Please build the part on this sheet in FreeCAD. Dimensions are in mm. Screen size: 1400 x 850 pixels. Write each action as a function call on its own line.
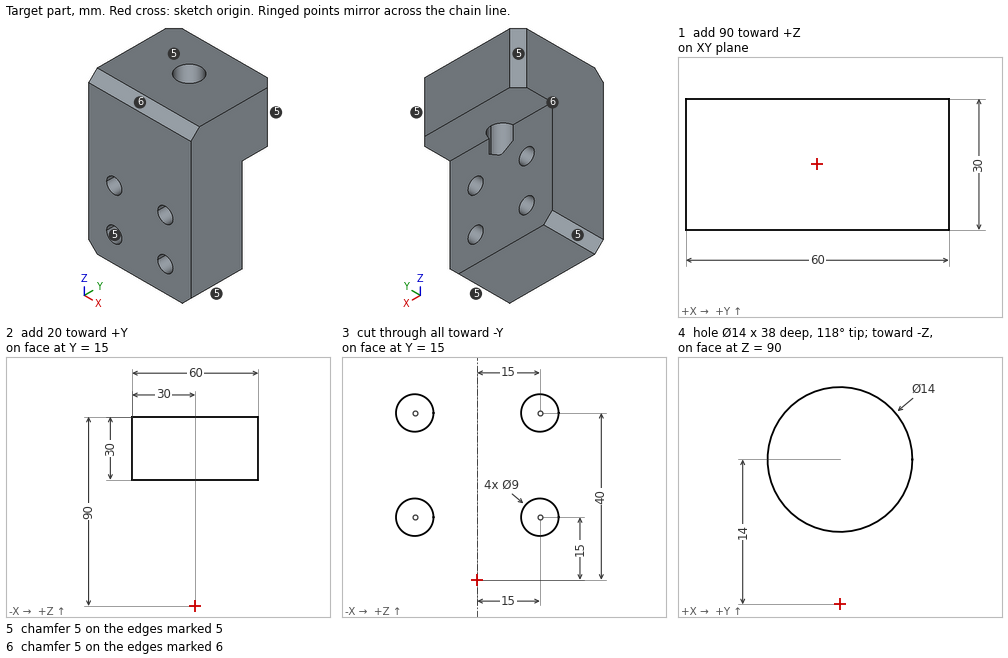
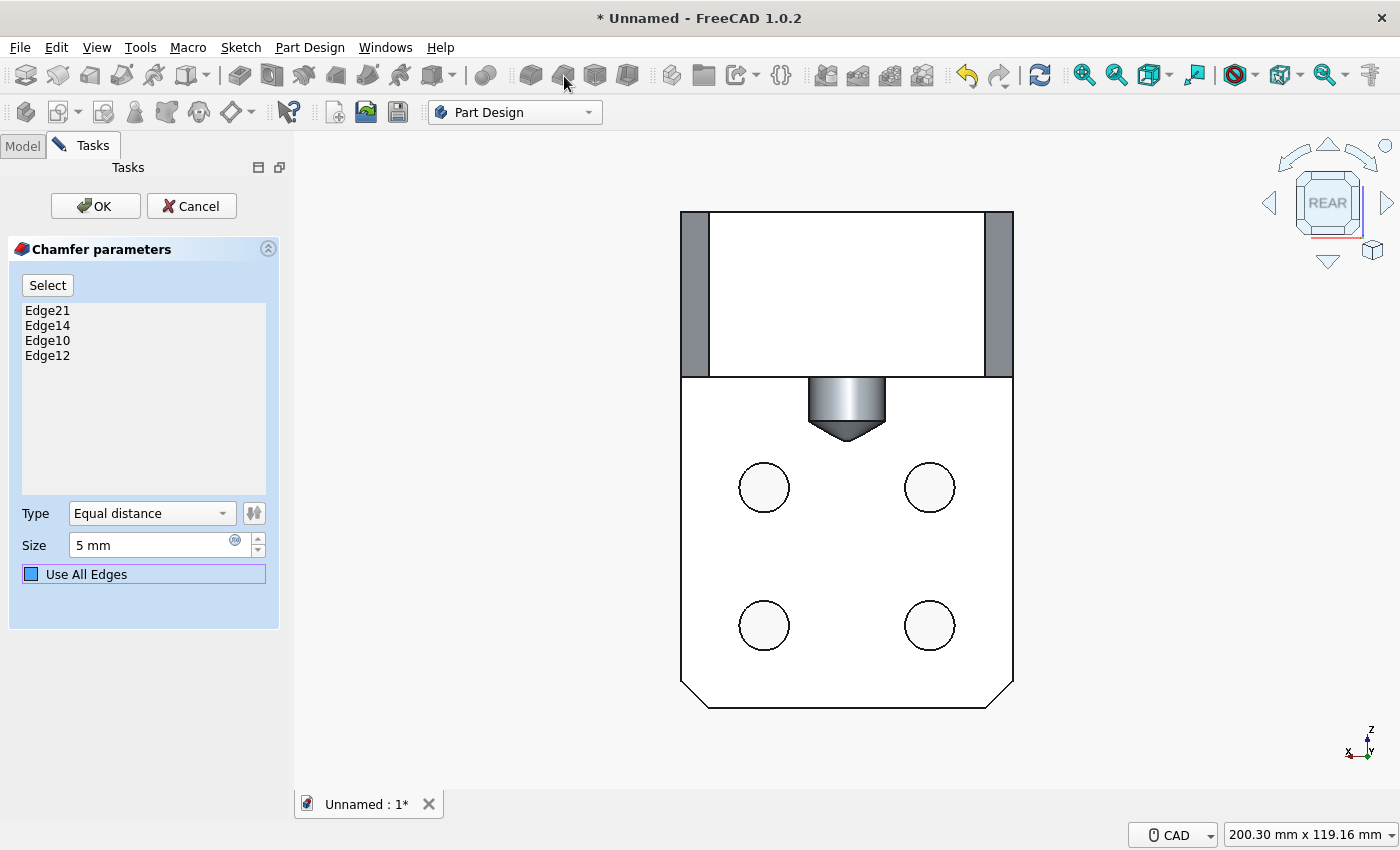
click(96, 206)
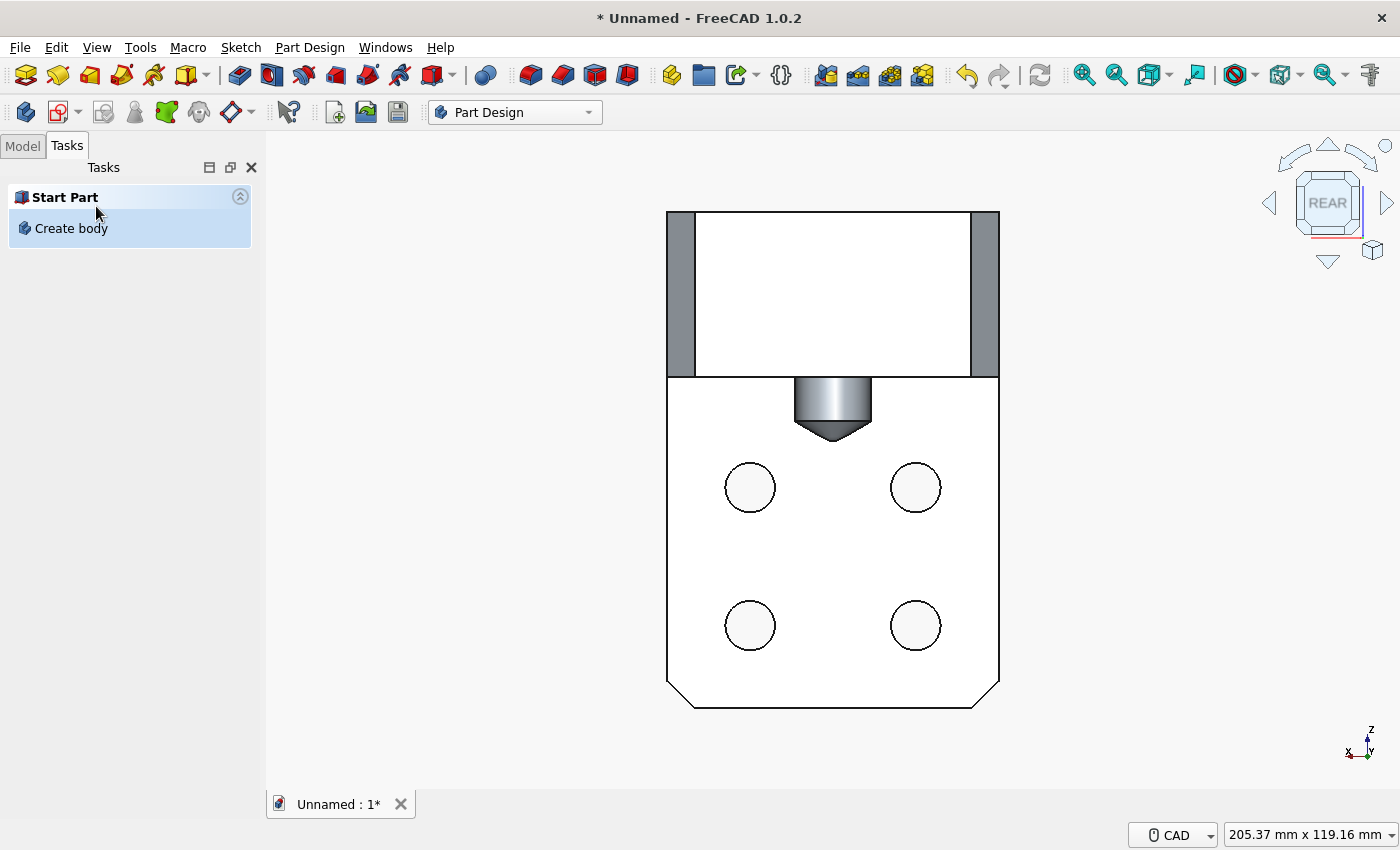
key(0)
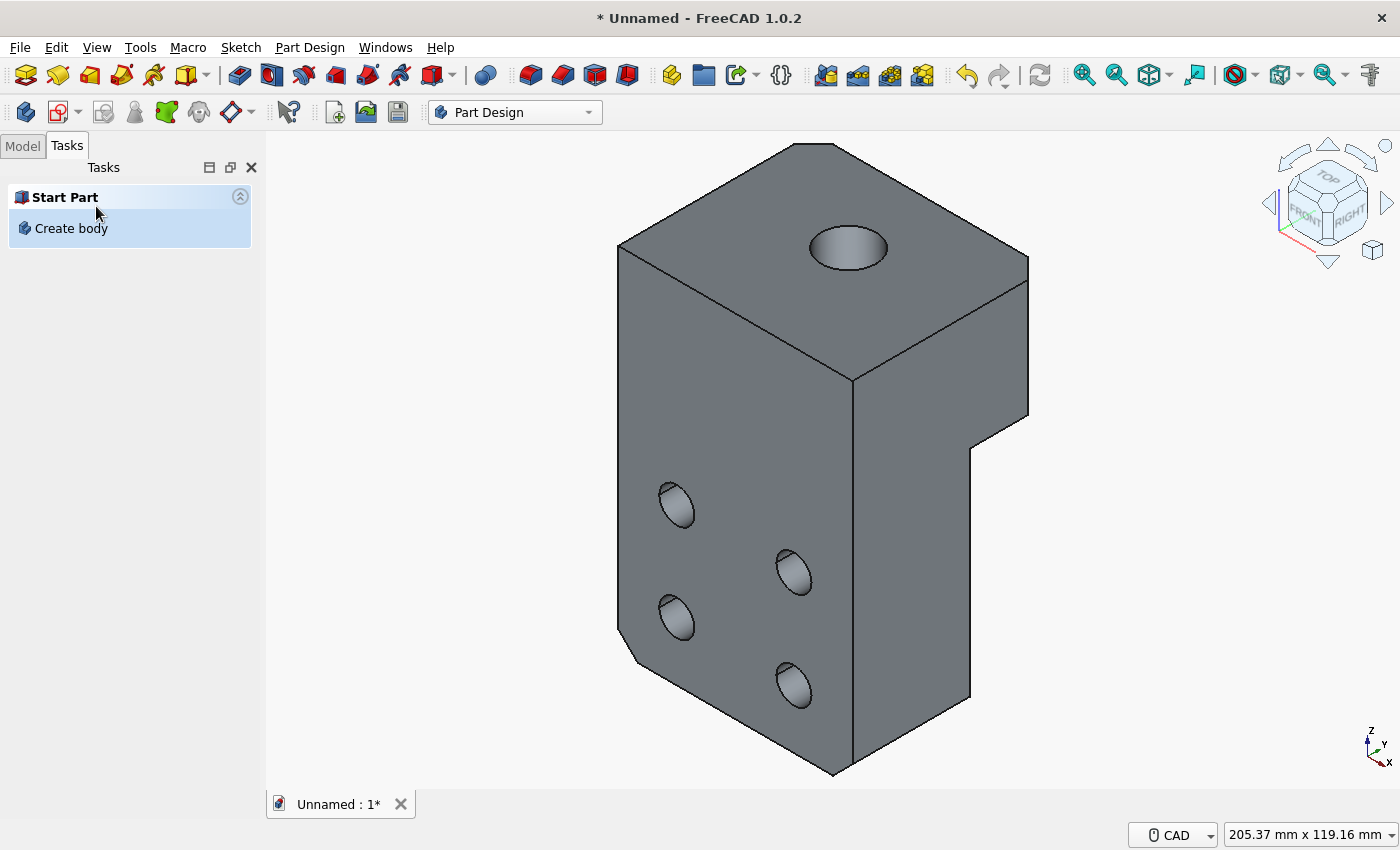
click(735, 312)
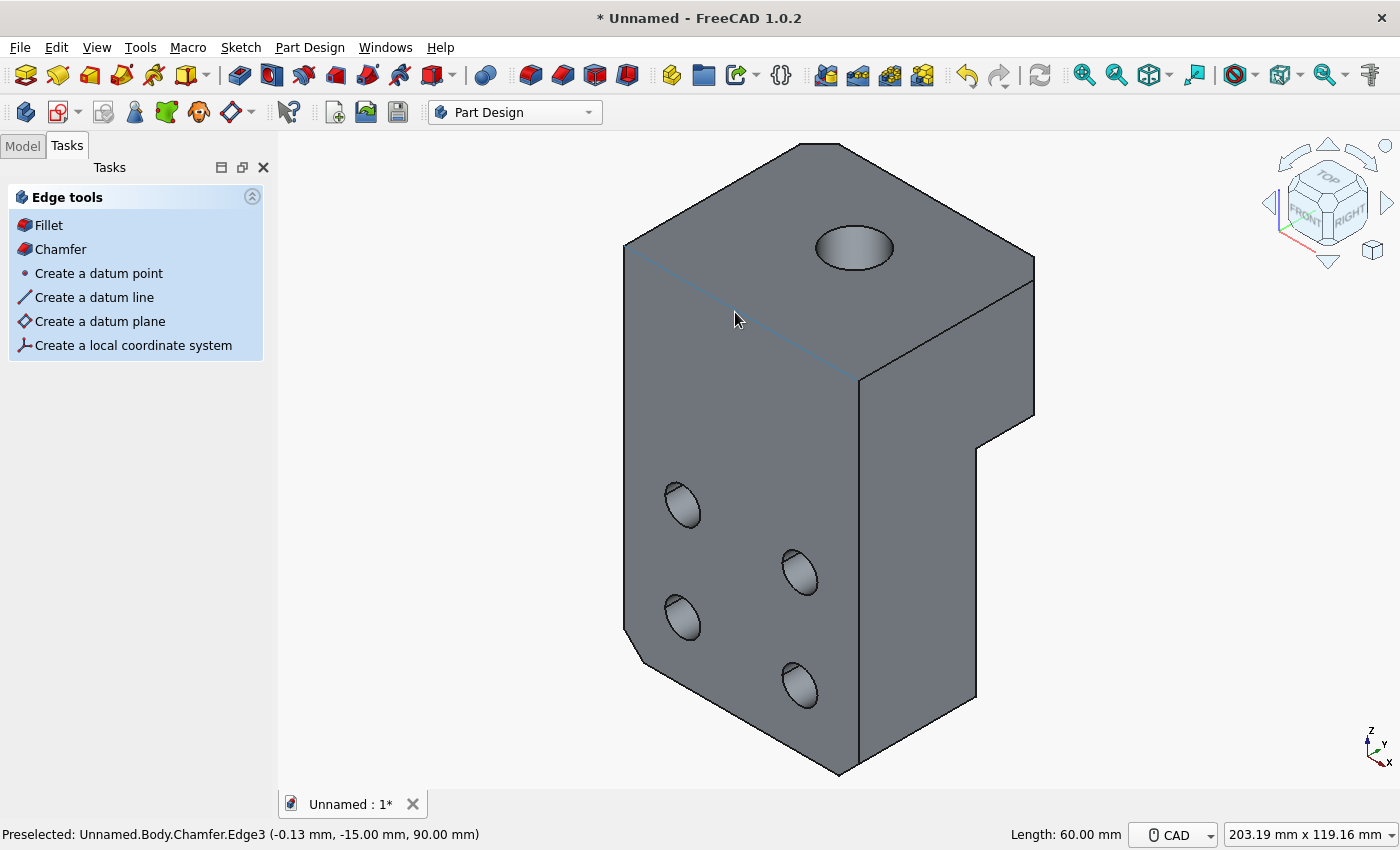
click(564, 76)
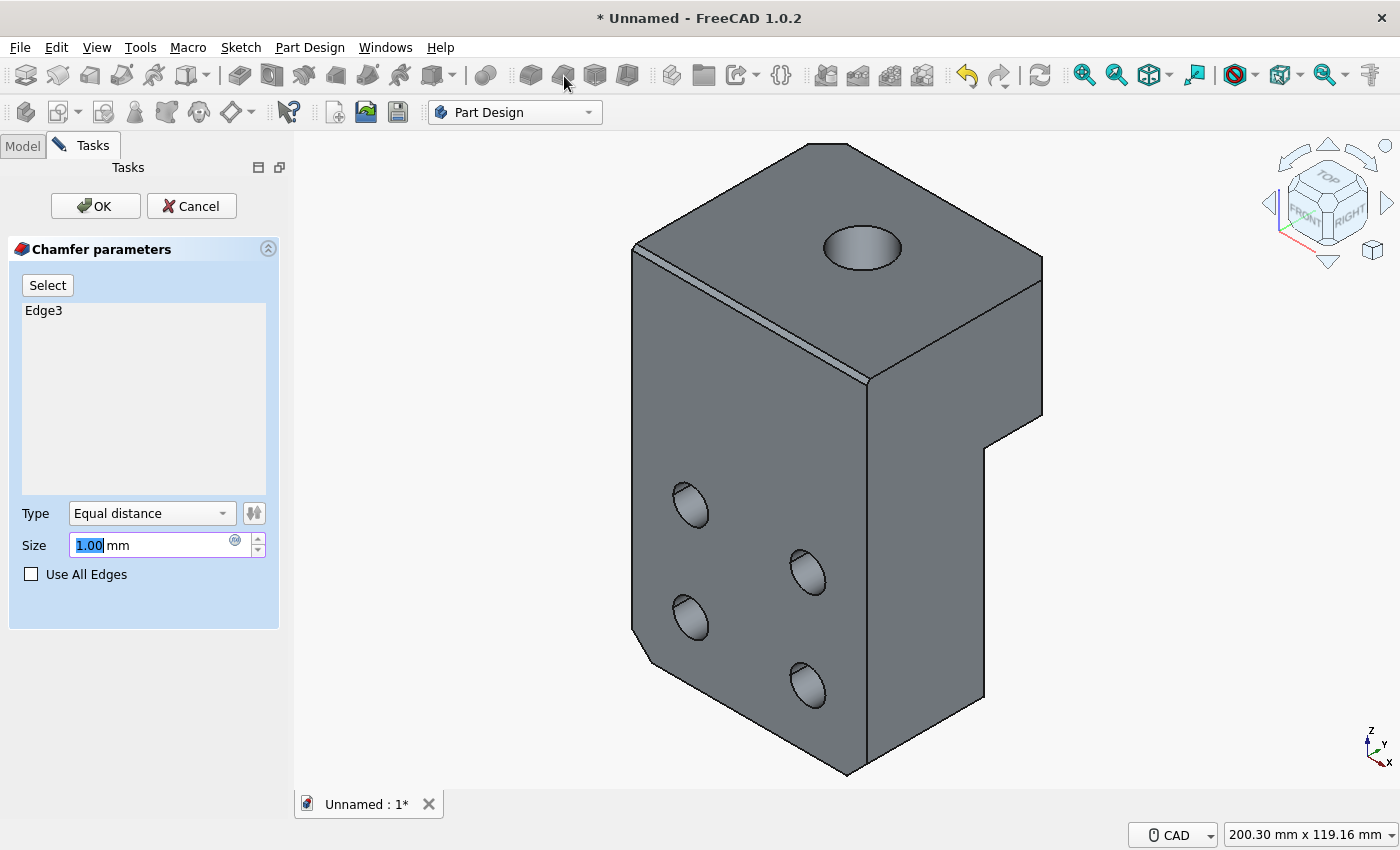
text(5)
key(Tab)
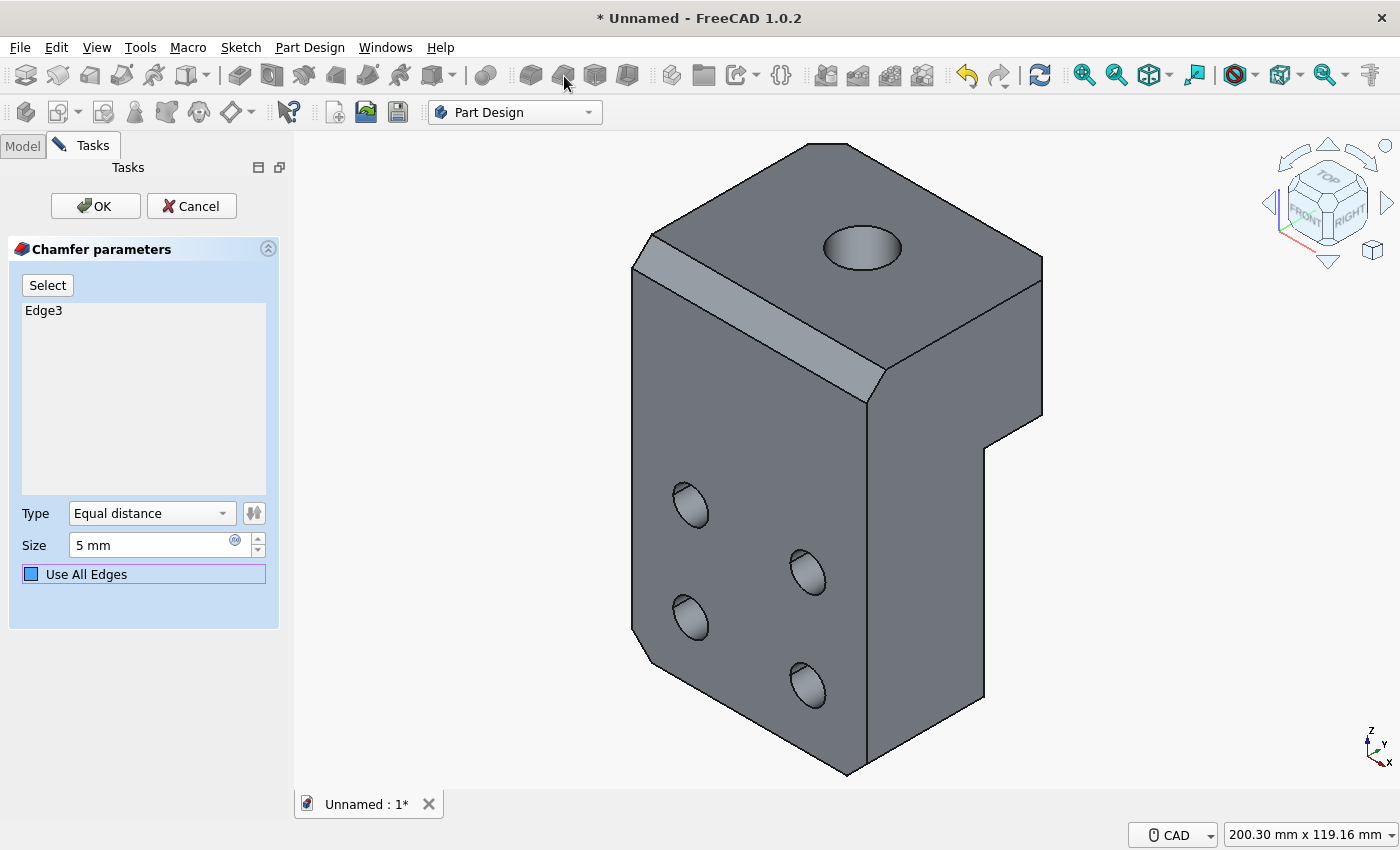
click(96, 206)